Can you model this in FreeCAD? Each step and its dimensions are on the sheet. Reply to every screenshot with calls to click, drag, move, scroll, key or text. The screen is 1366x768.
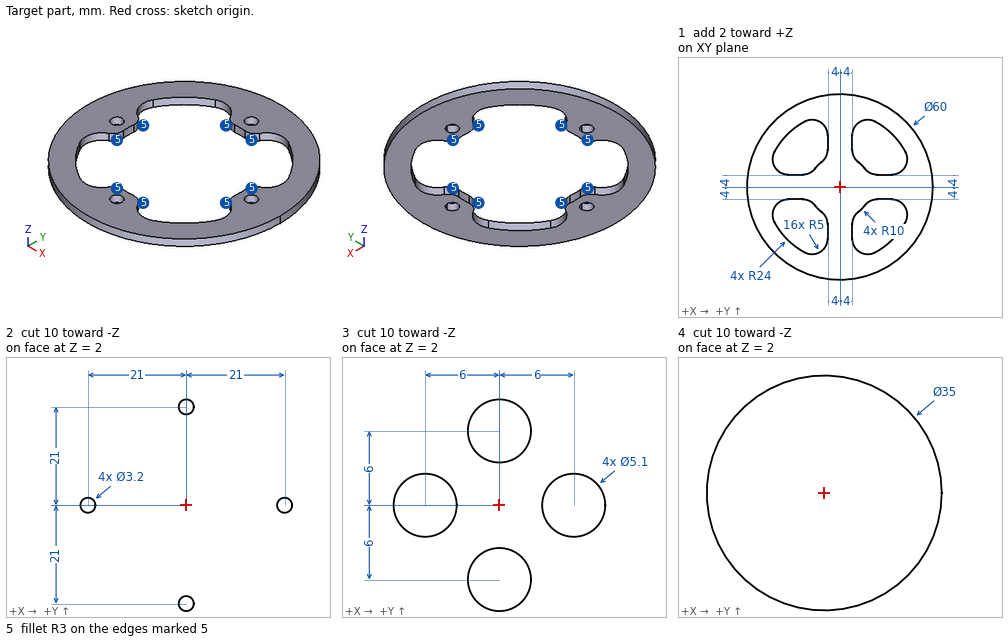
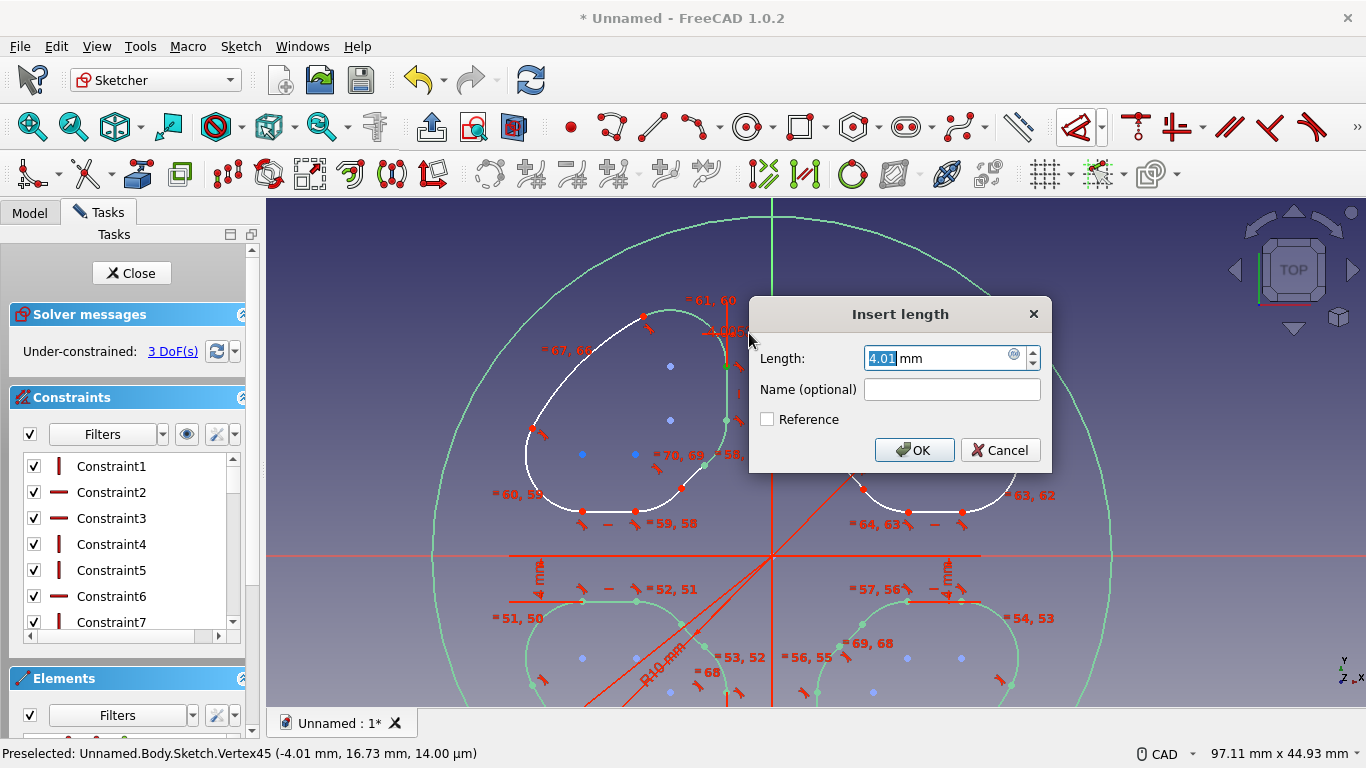
text(4)
key(Return)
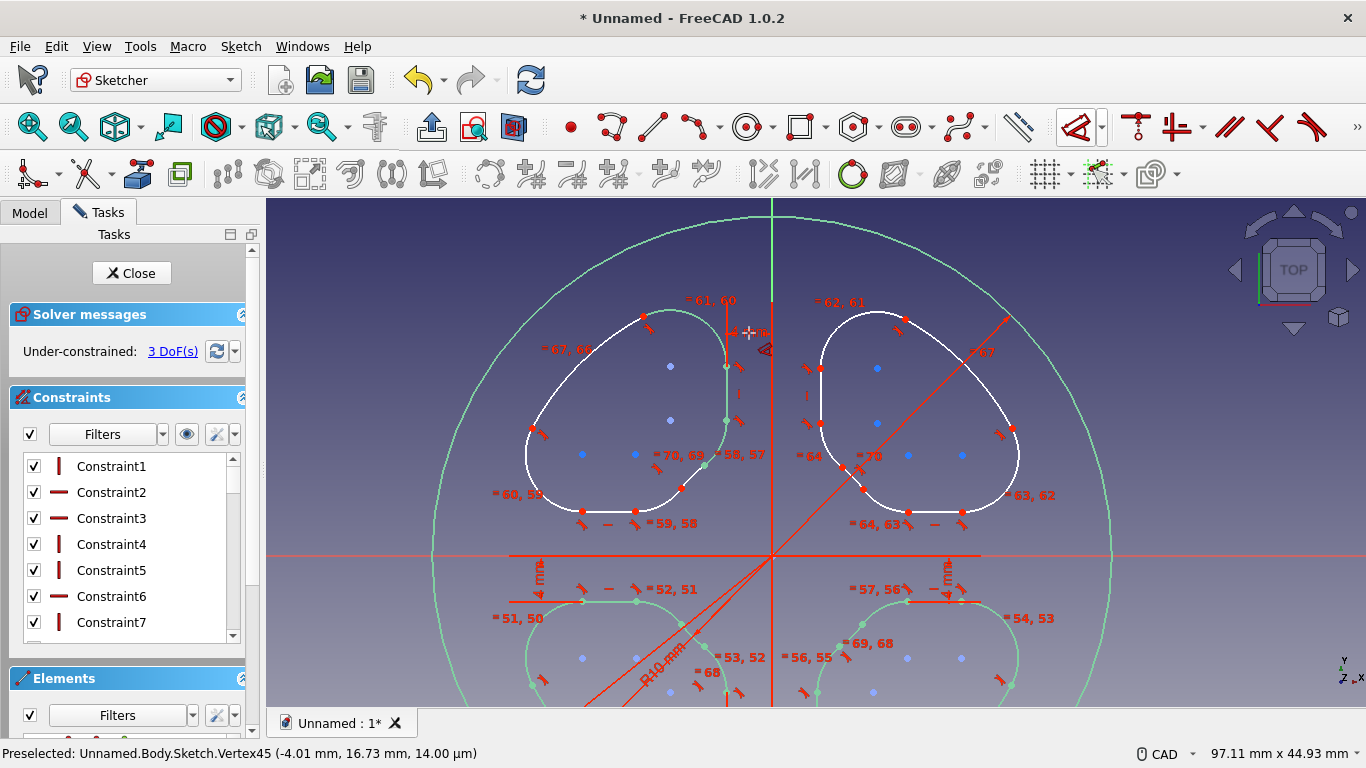
click(636, 512)
click(602, 534)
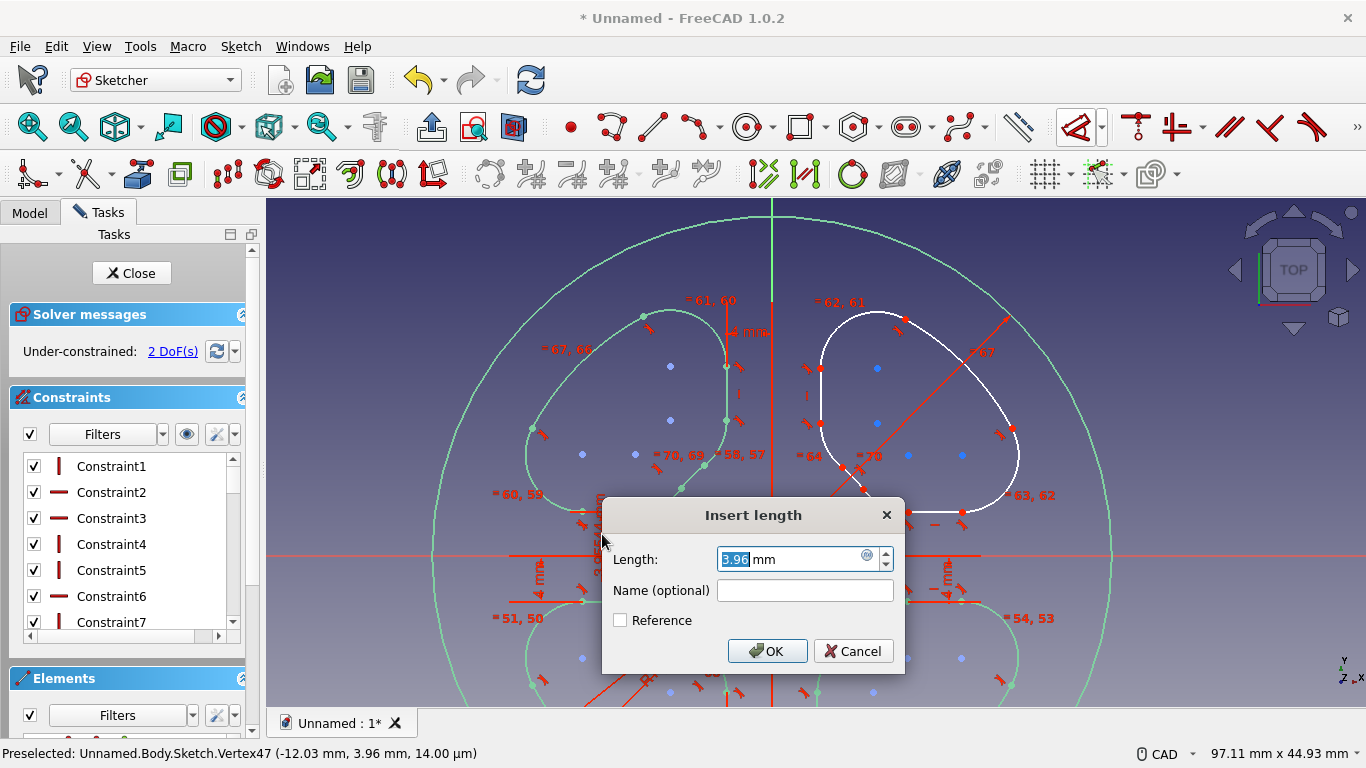
text(4)
key(Return)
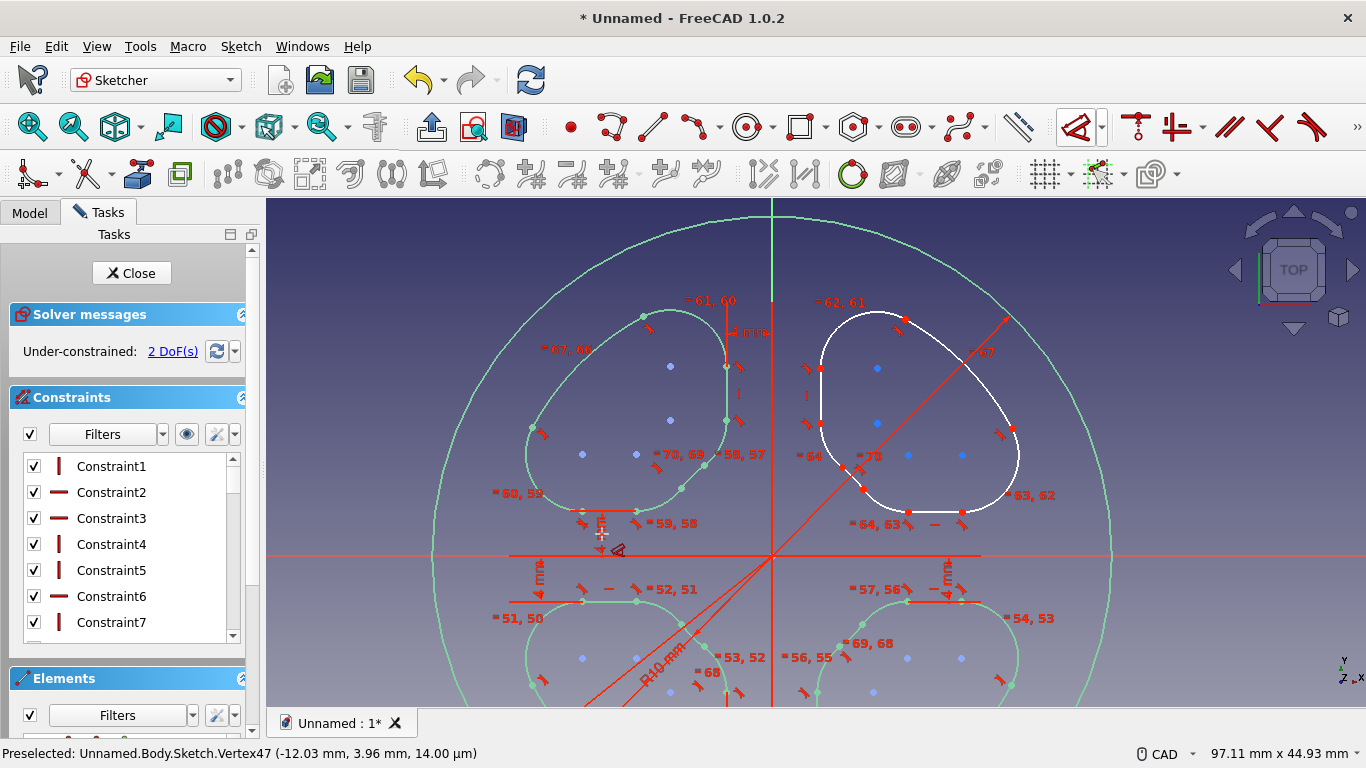
click(821, 423)
click(796, 389)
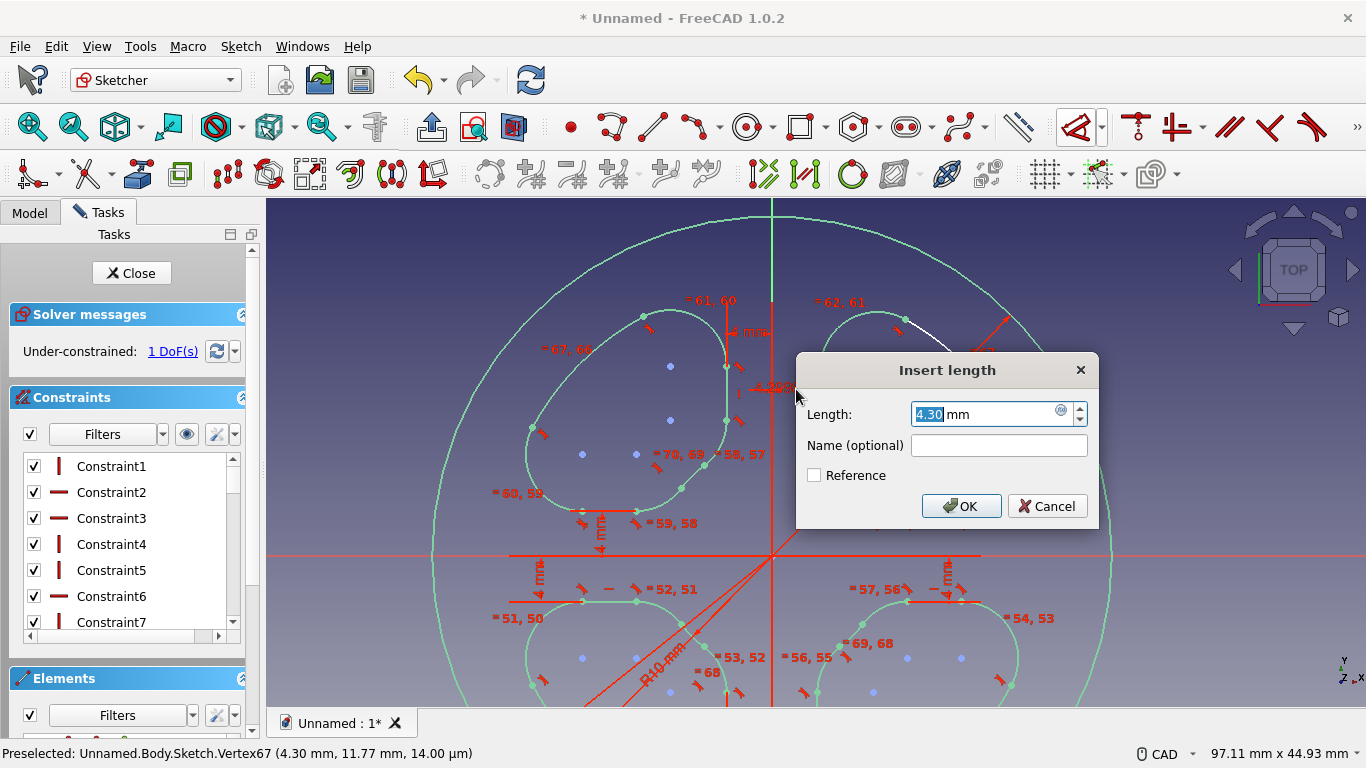
text(4)
key(Return)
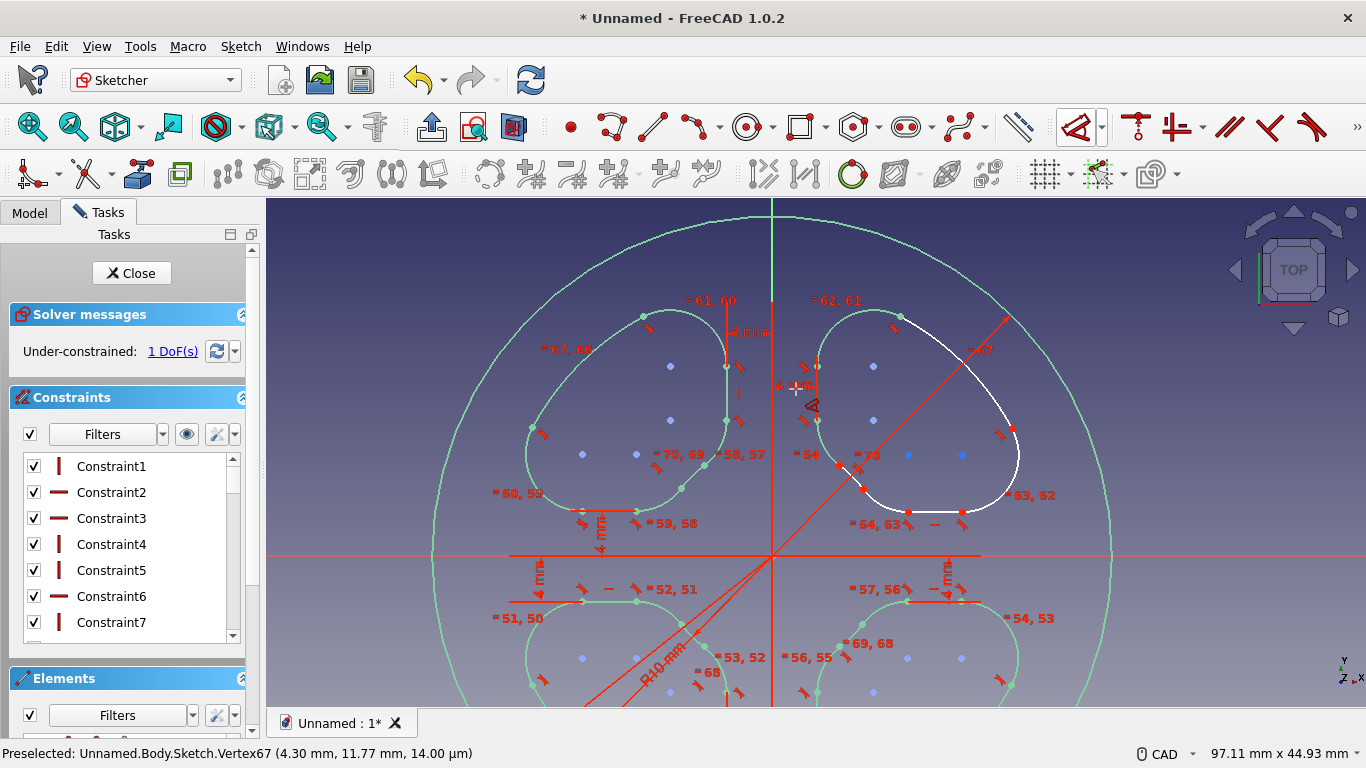
click(962, 512)
click(996, 534)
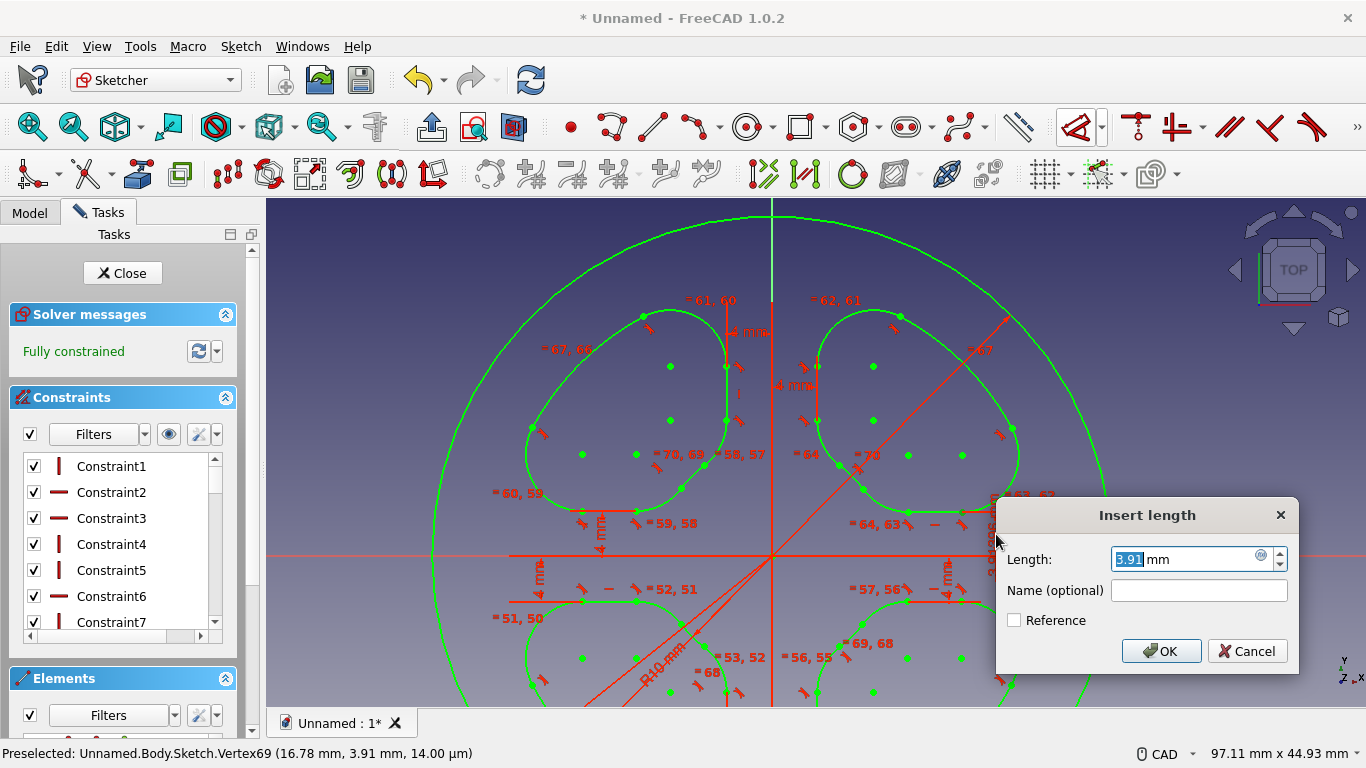
text(4)
key(Return)
key(Escape)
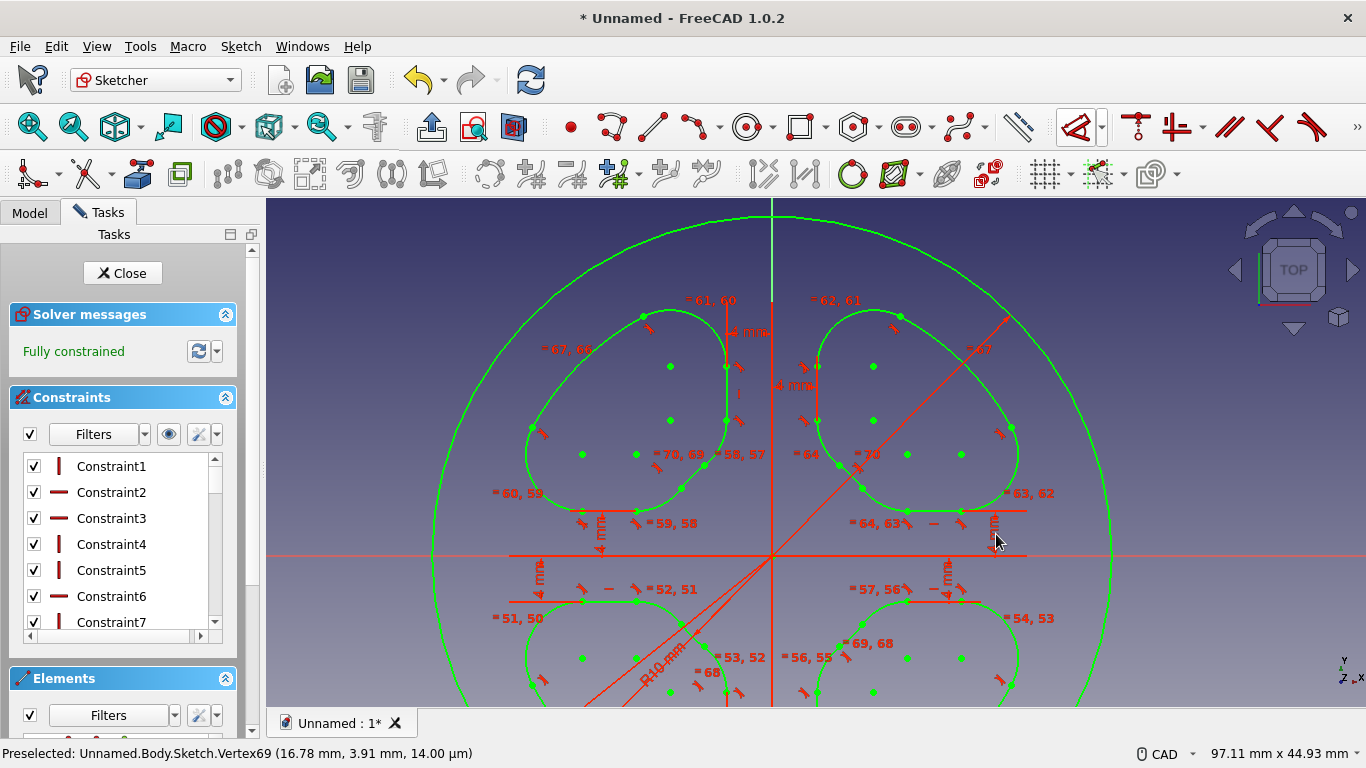
click(123, 273)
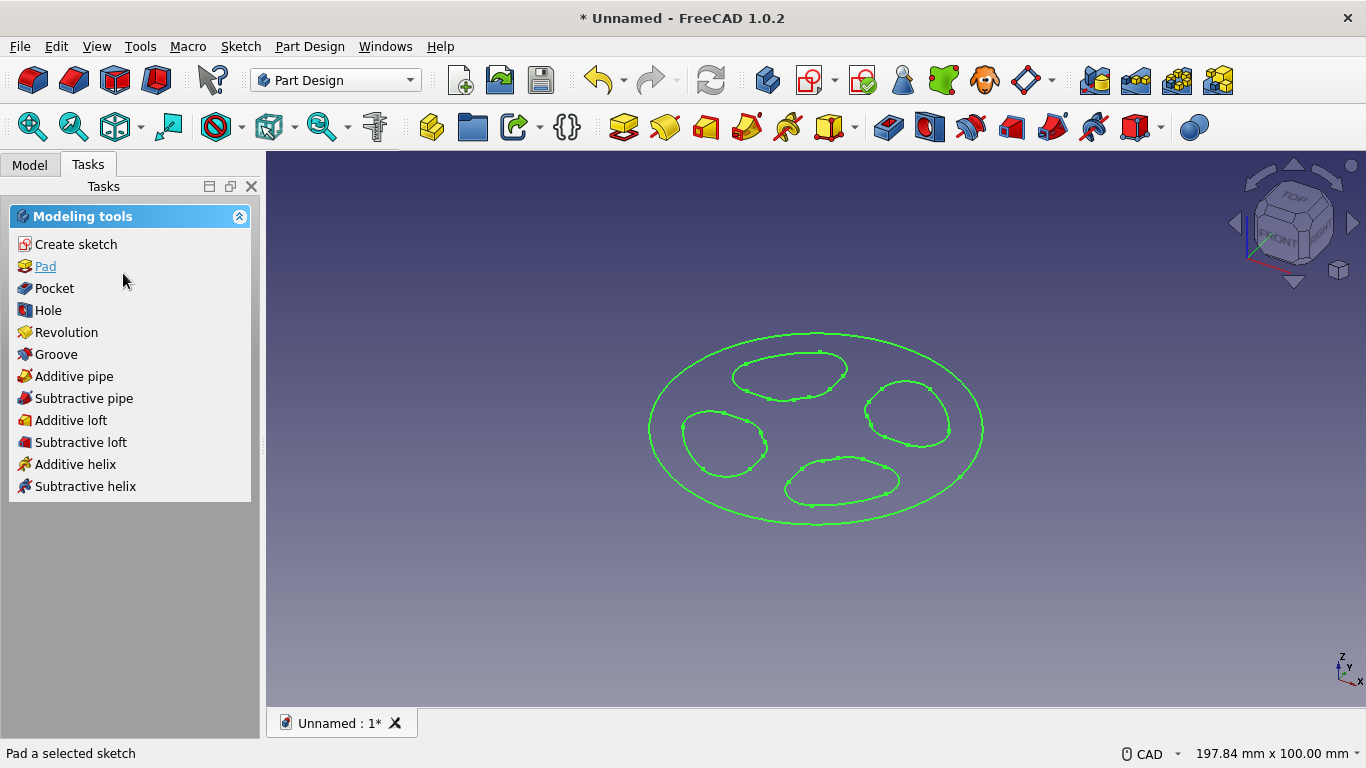
click(624, 128)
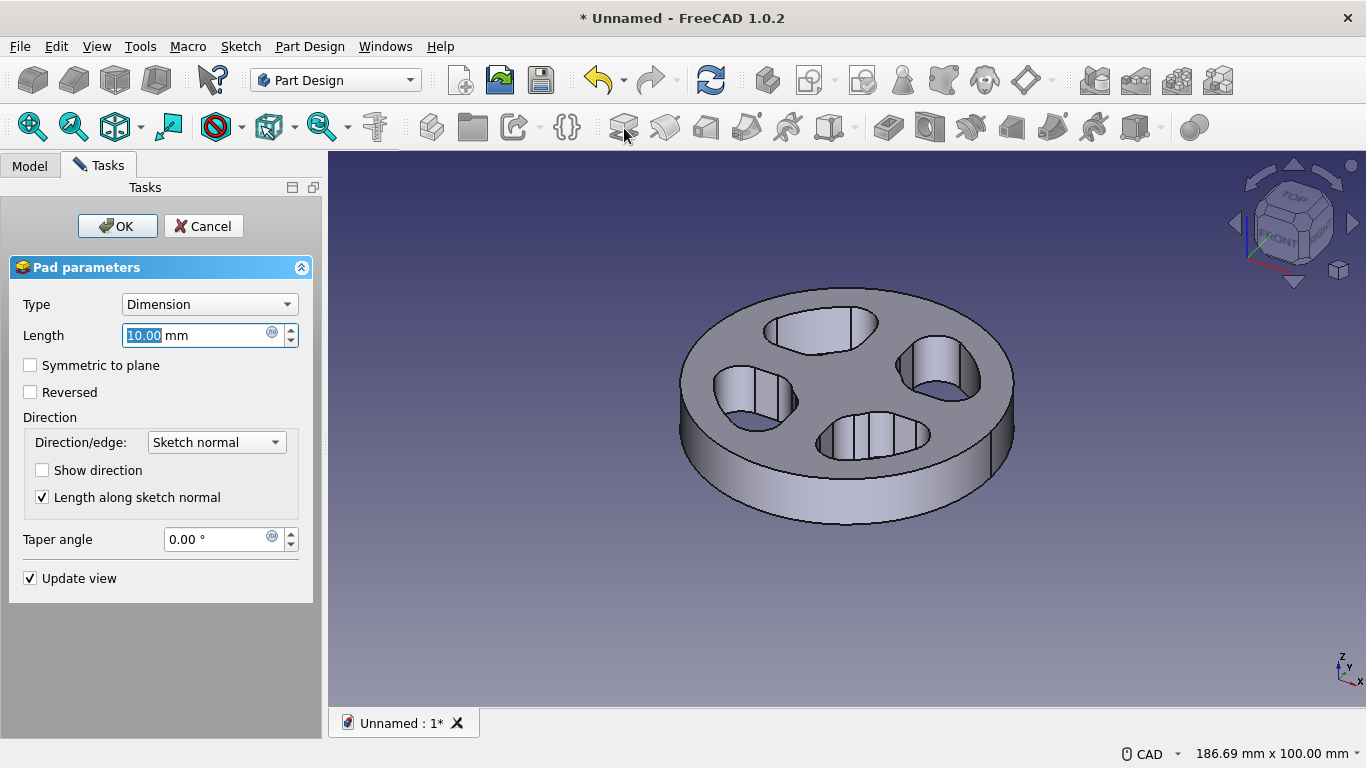
text(2)
key(Tab)